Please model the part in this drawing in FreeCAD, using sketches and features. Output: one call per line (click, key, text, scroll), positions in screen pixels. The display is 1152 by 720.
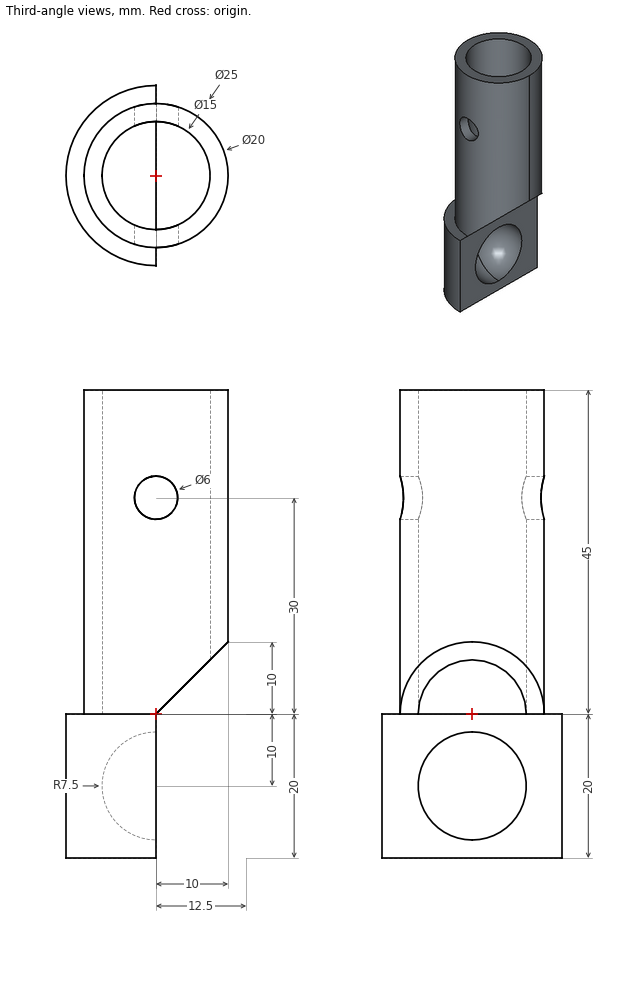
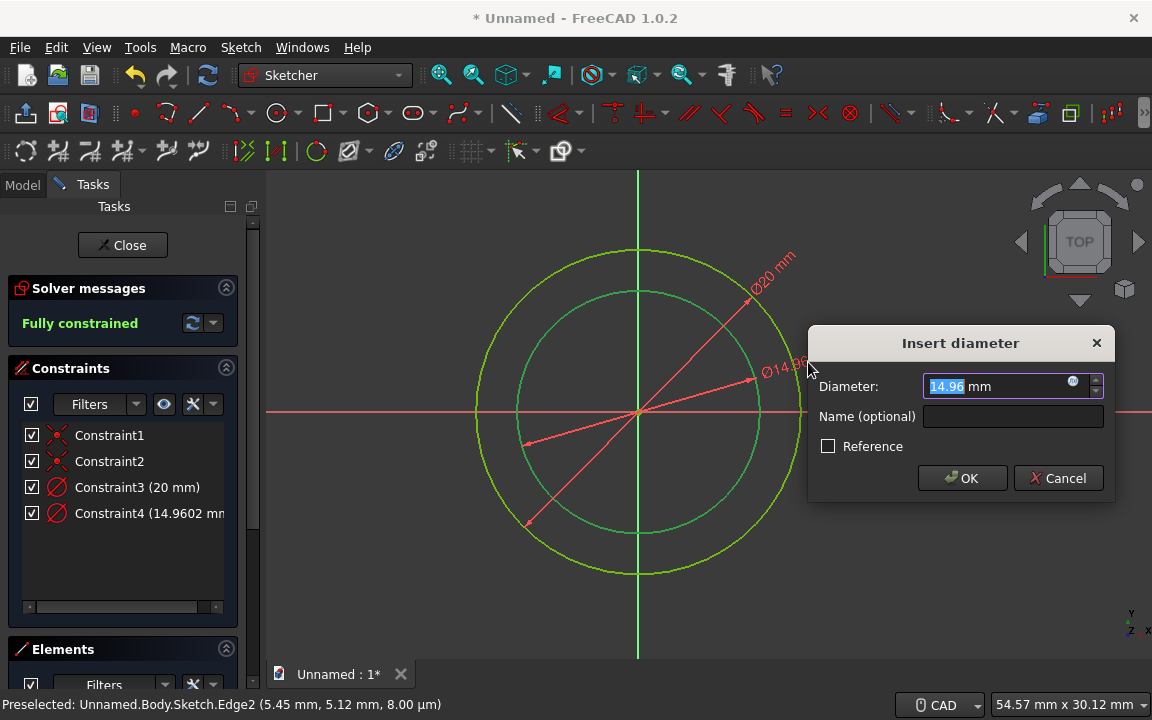
text(15)
key(Return)
key(Escape)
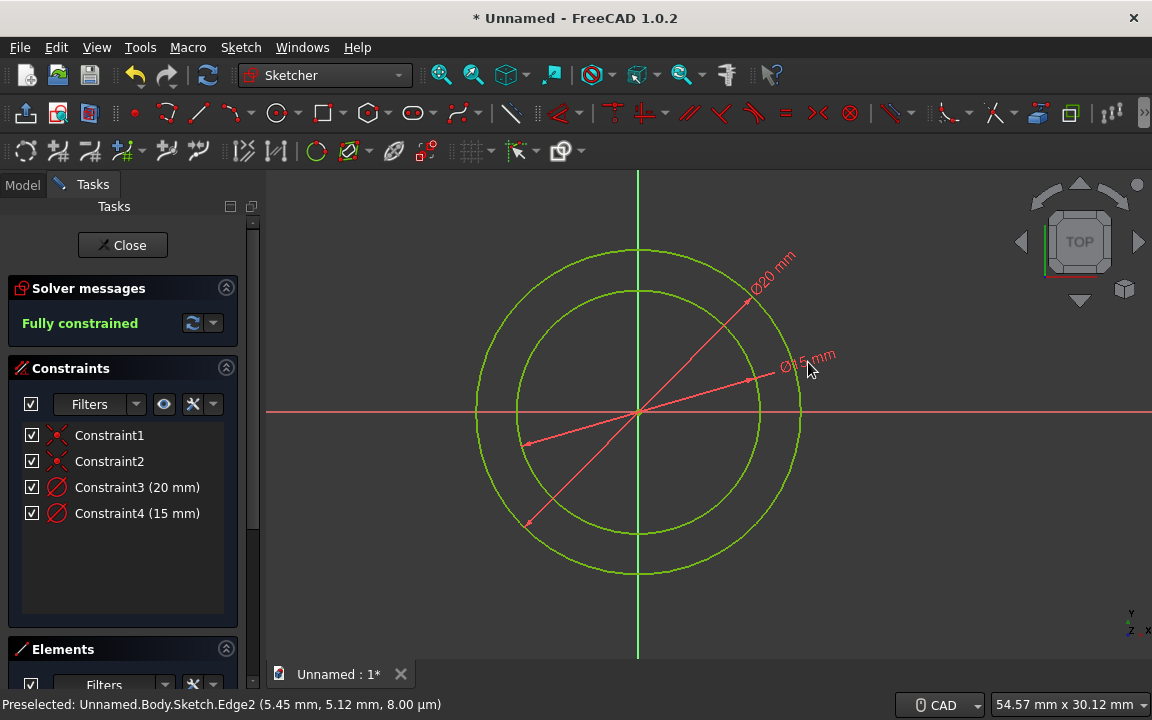
click(123, 245)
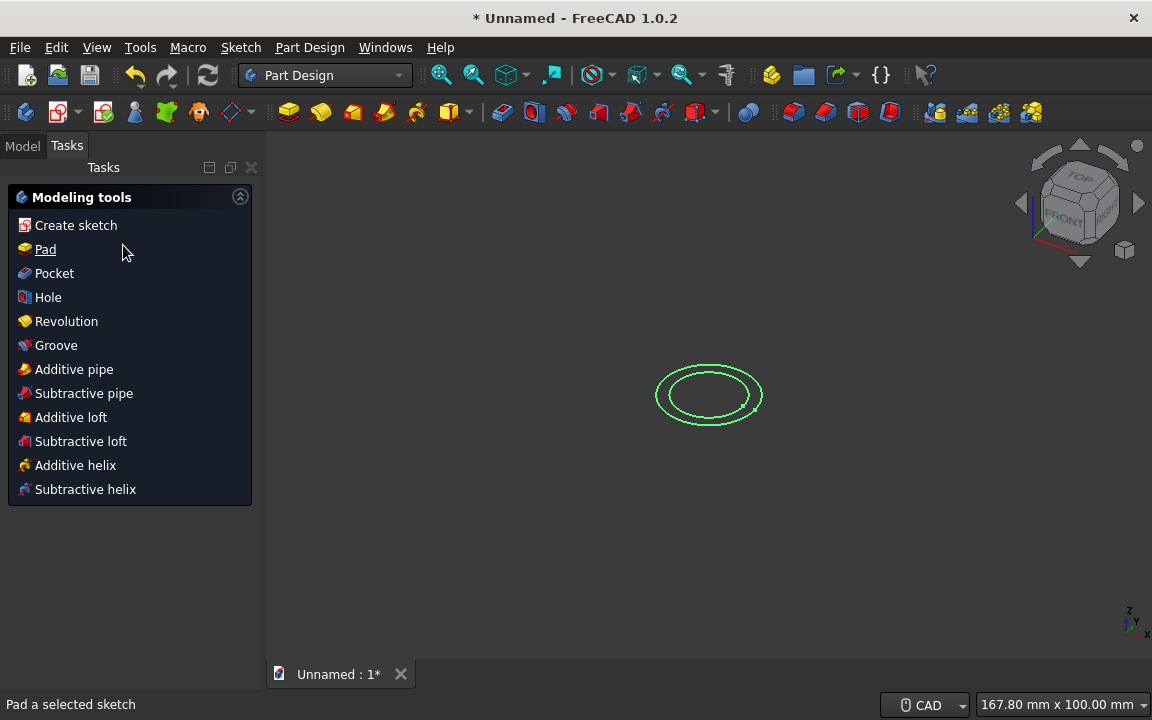
click(290, 112)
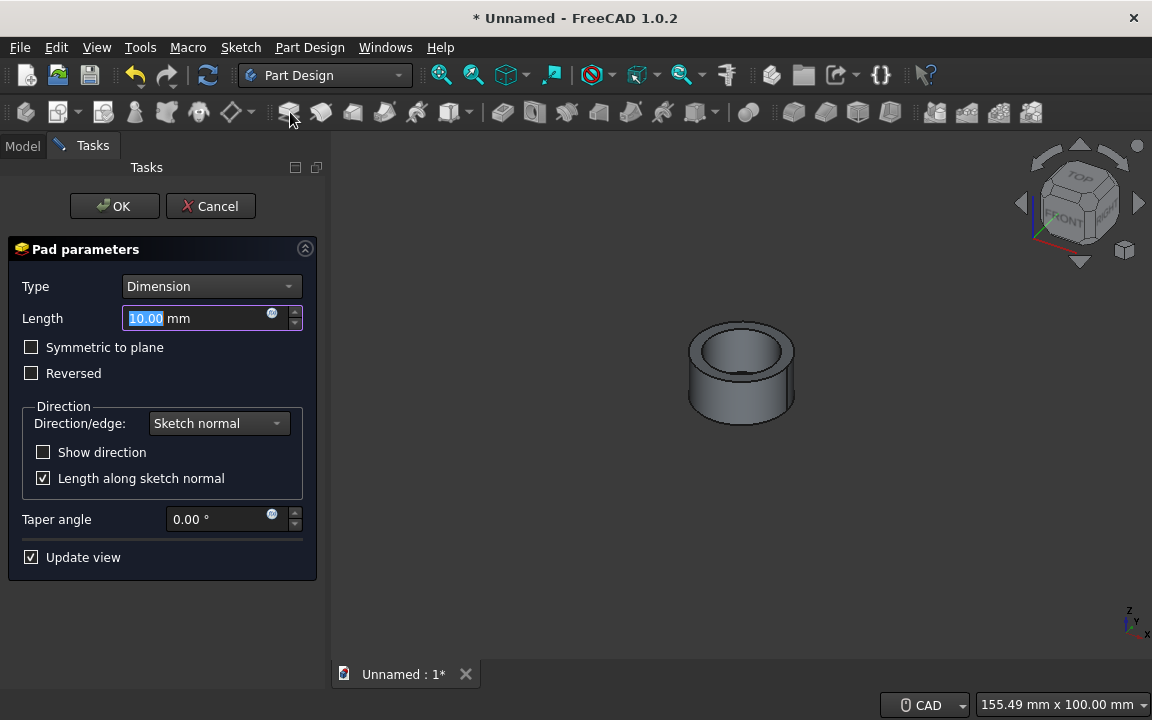
text(45)
key(Tab)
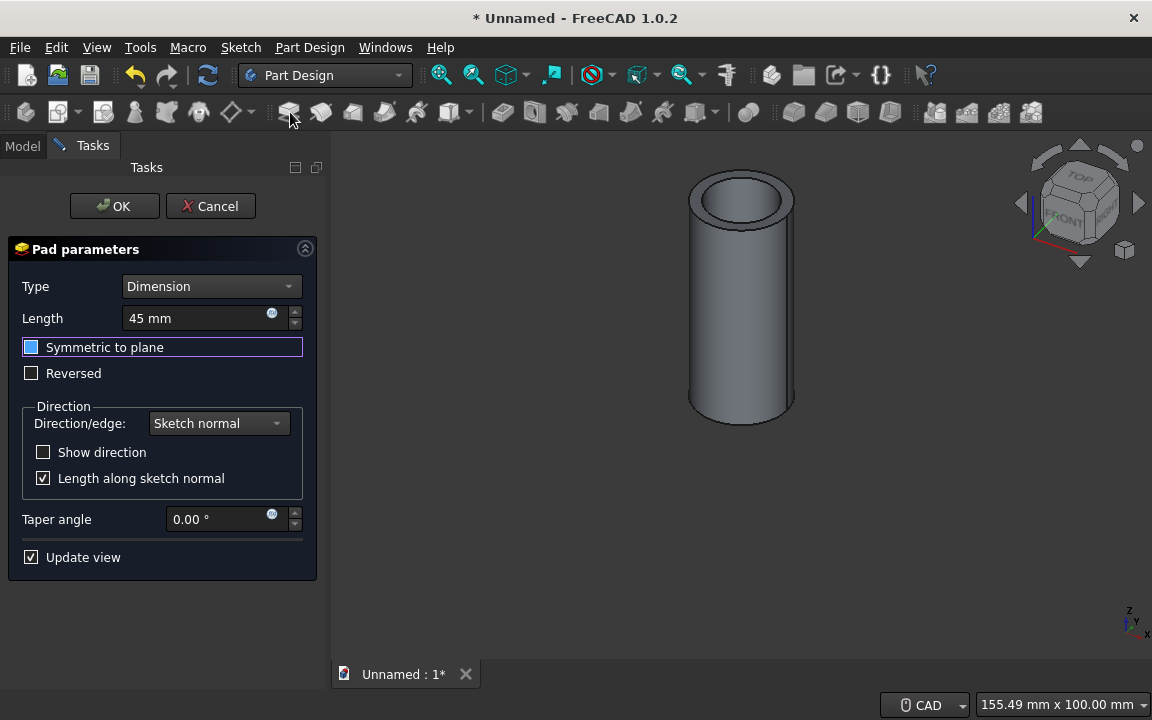
click(115, 206)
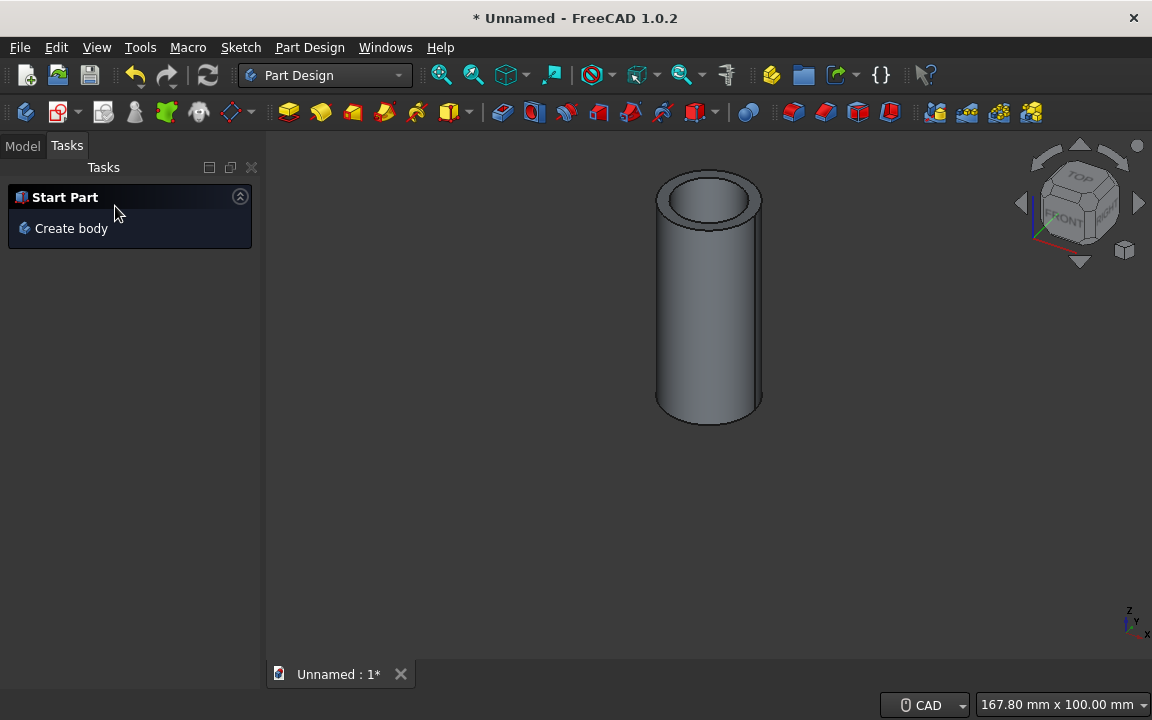
click(58, 112)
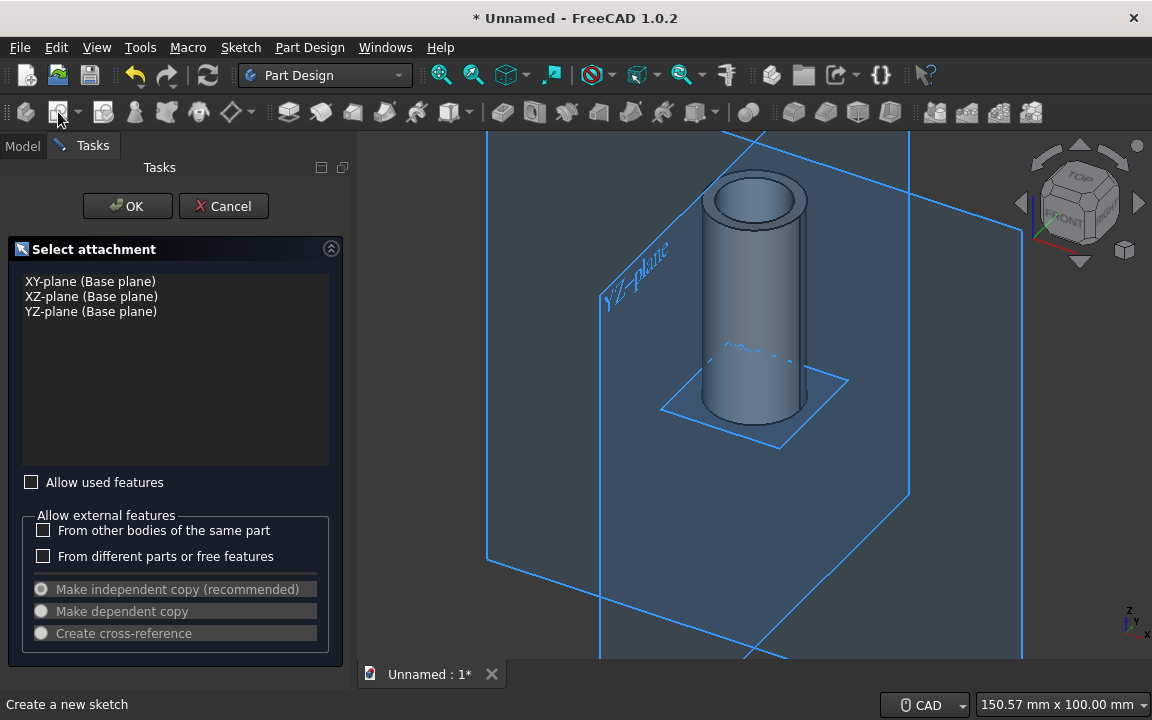
click(82, 296)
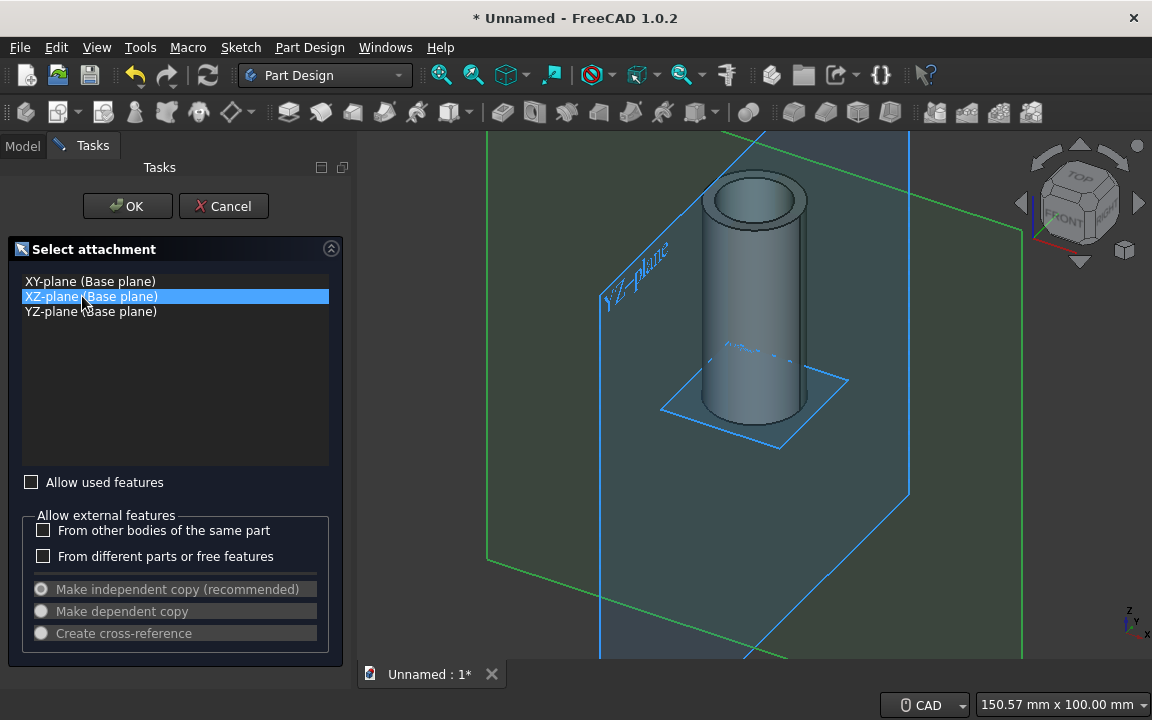
click(128, 206)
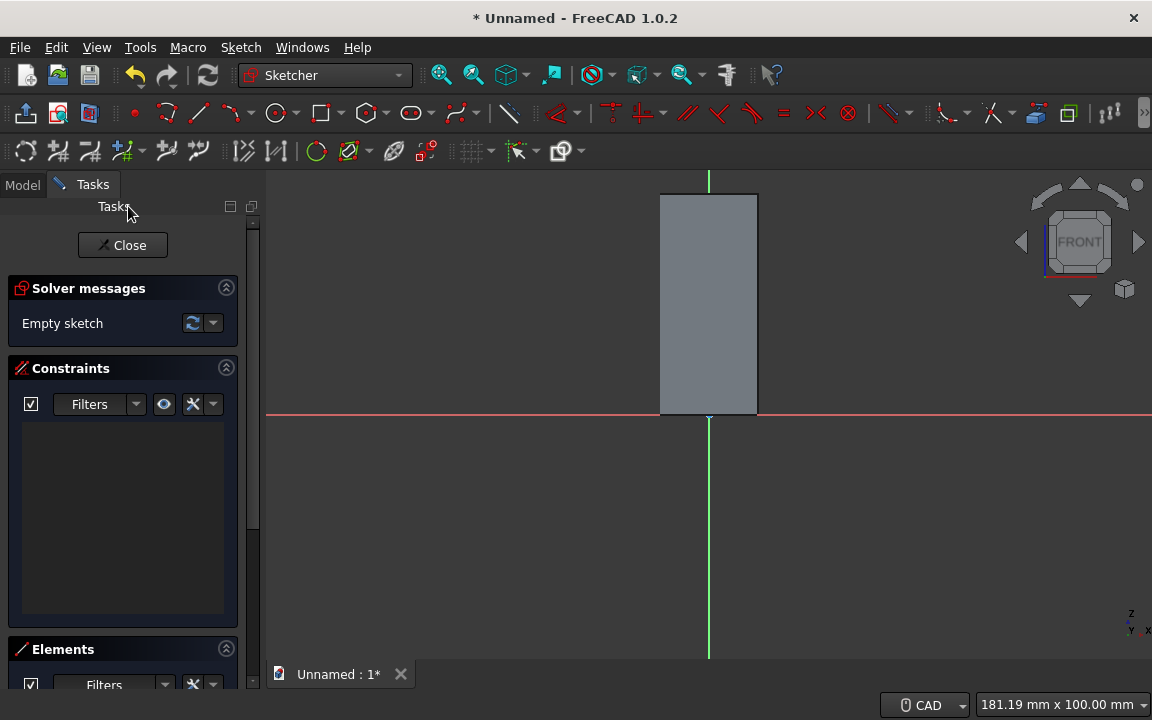
click(90, 114)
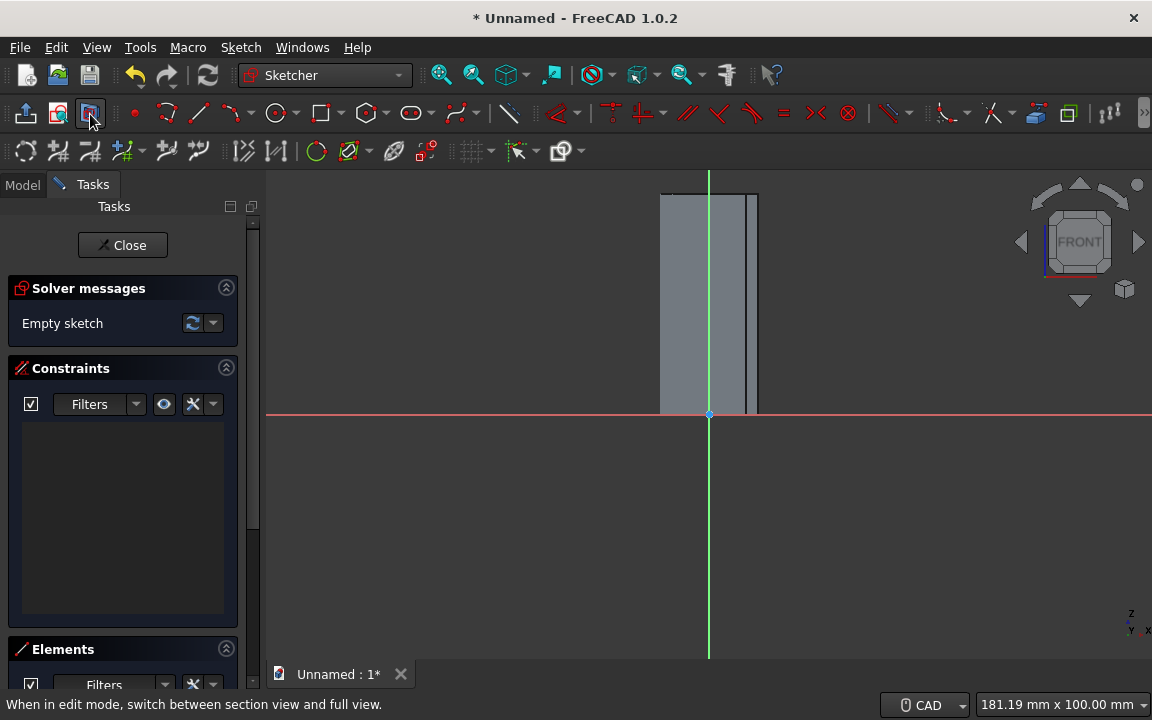
scroll(716, 253, up, 12)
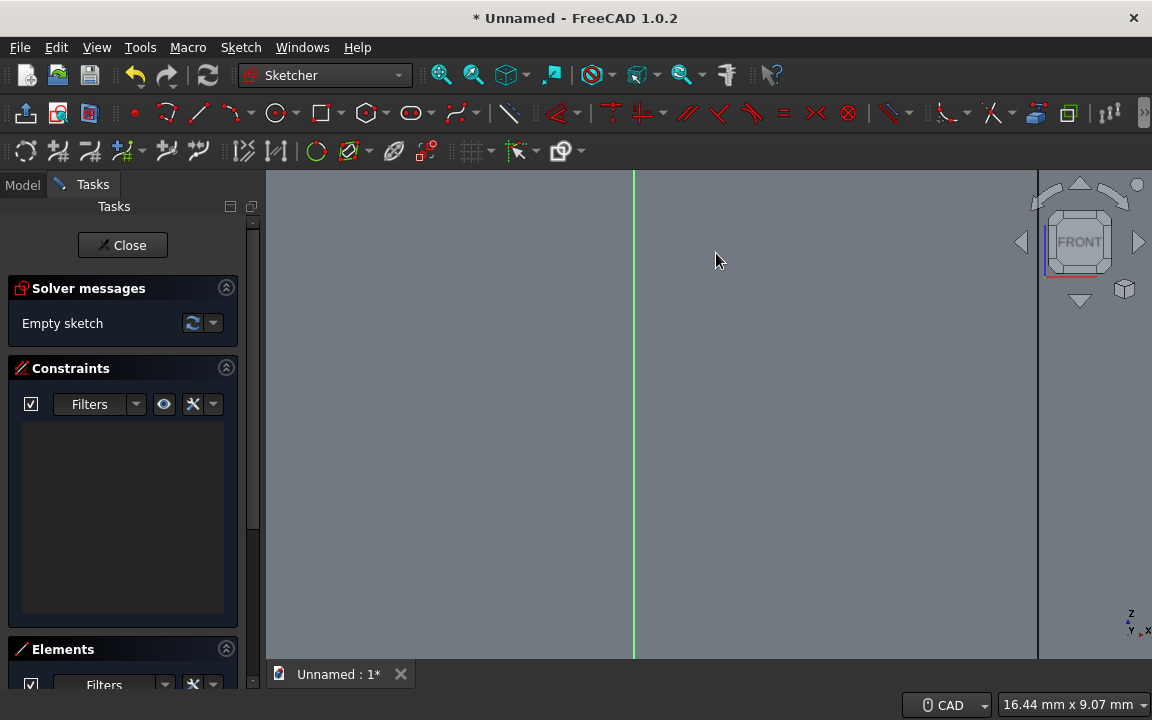
click(276, 114)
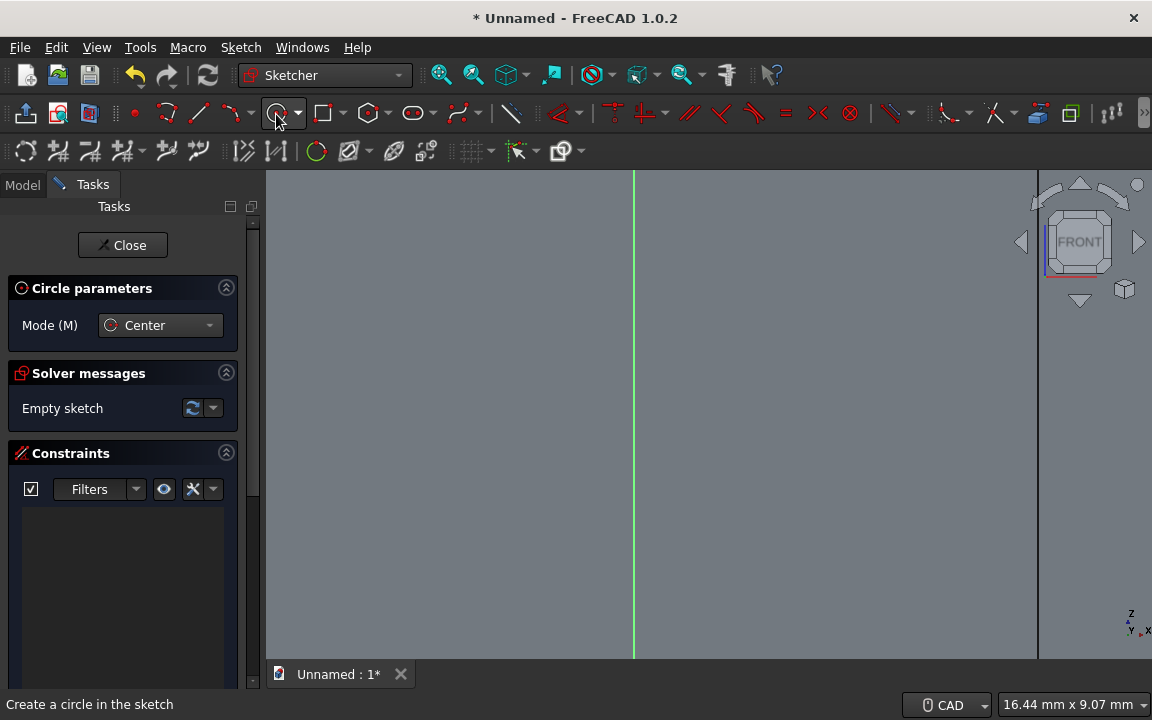
click(634, 414)
click(748, 300)
key(Escape)